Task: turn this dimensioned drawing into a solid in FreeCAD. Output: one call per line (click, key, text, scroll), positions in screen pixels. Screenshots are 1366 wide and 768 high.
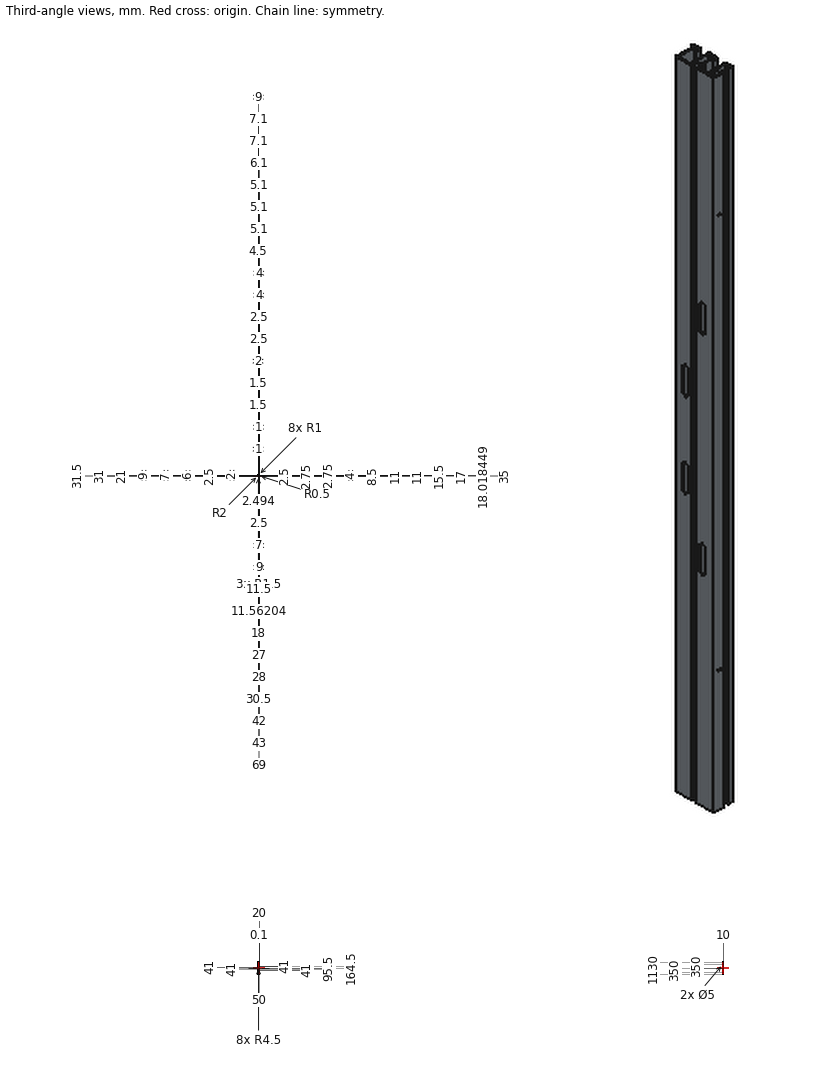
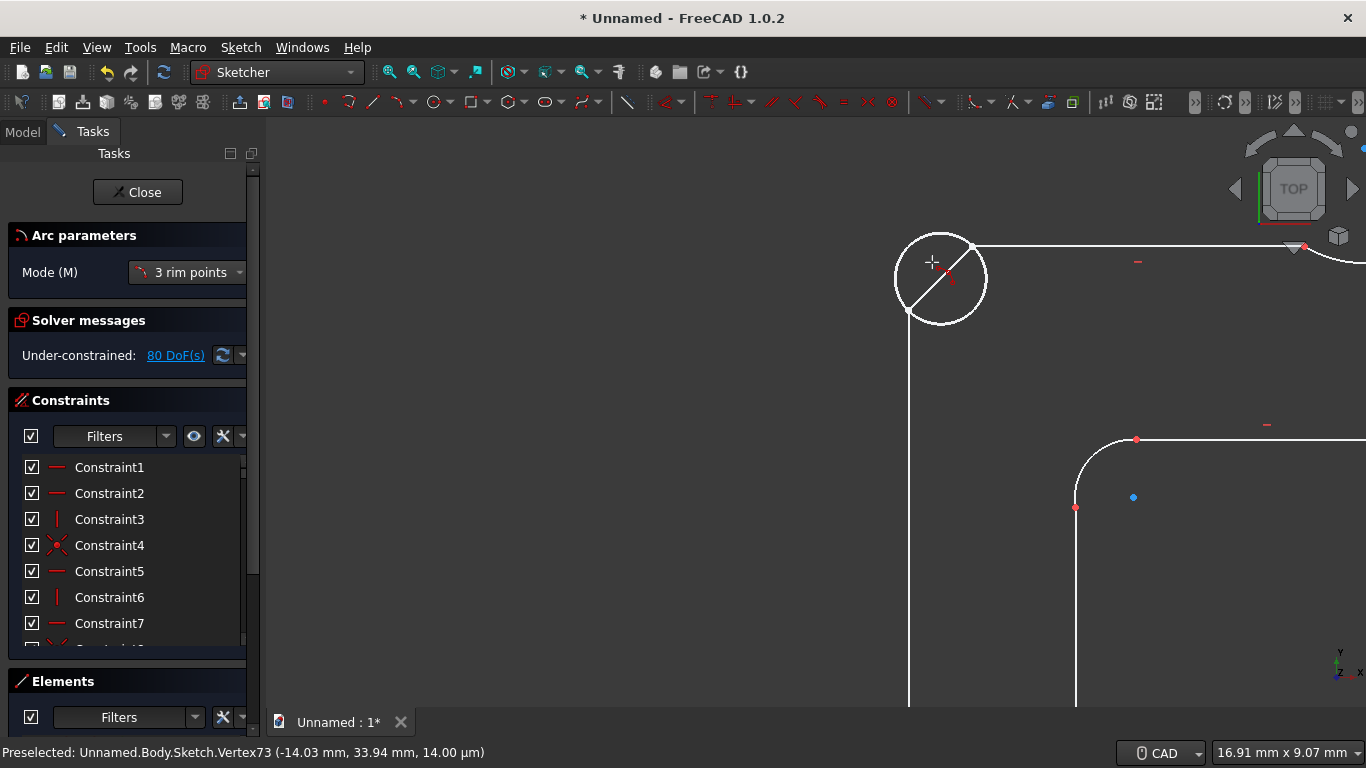
click(929, 261)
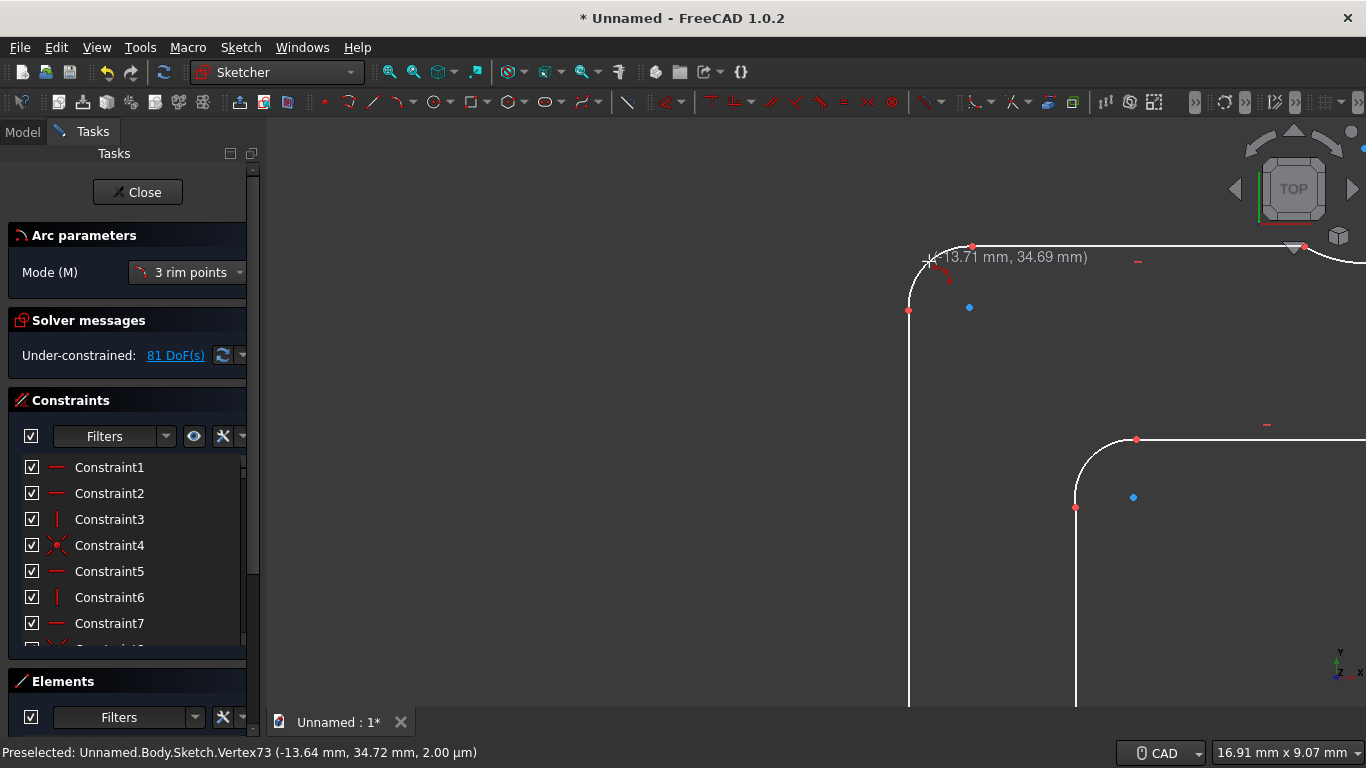
scroll(936, 260, down, 10)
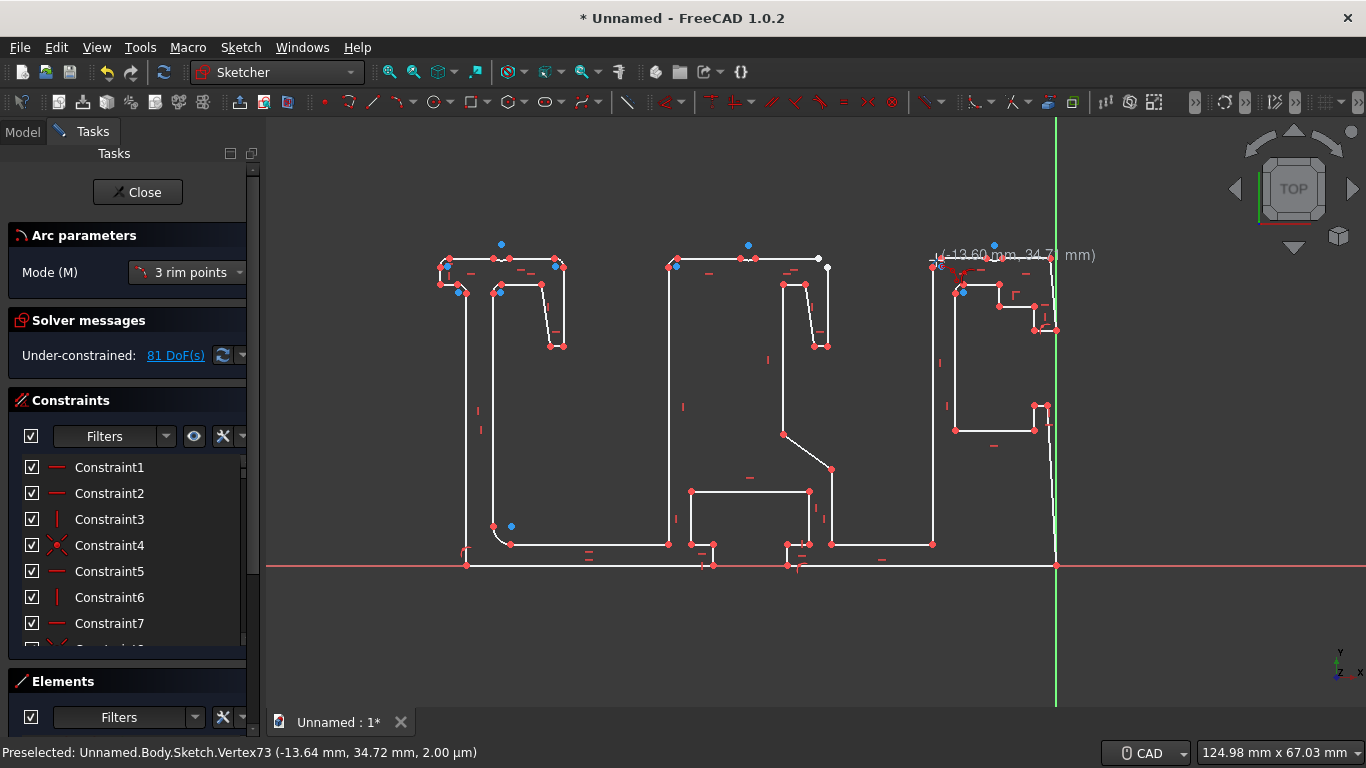
scroll(827, 267, up, 2)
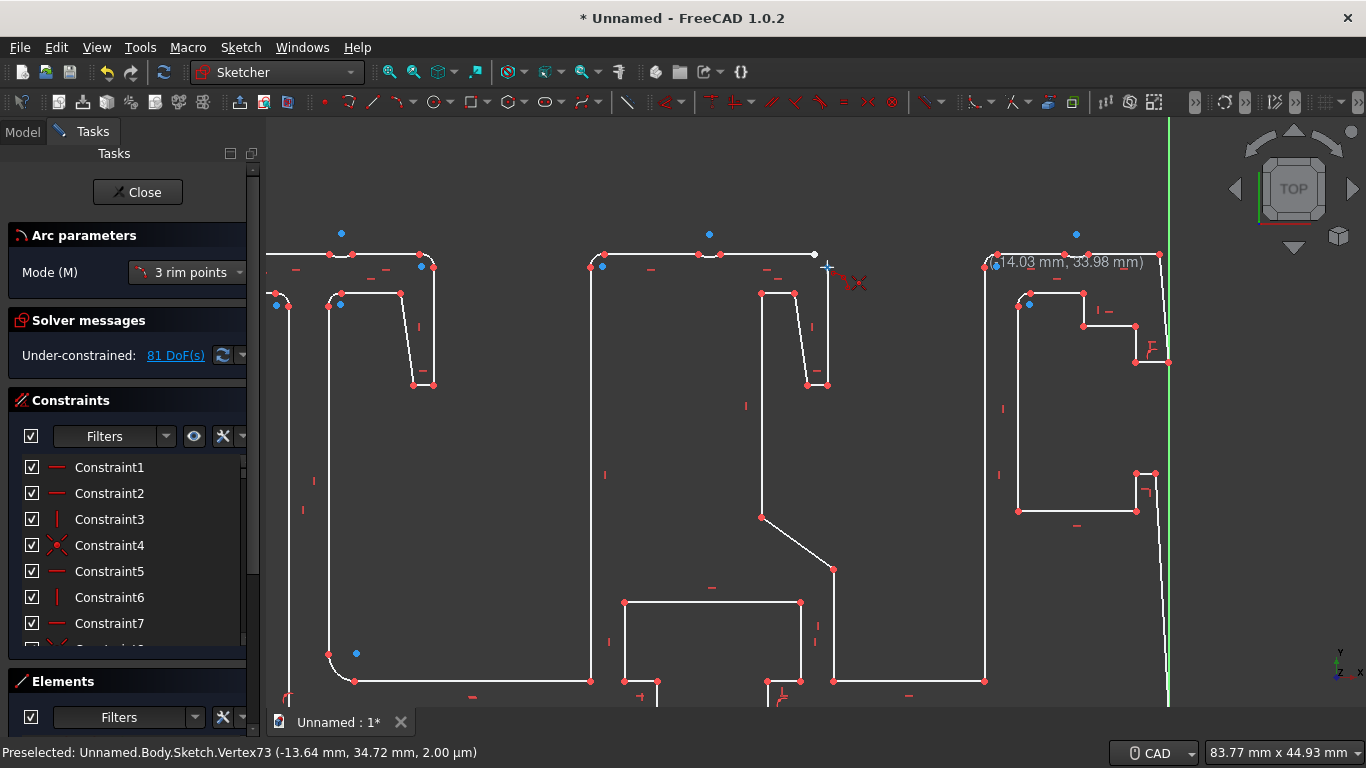
click(828, 267)
click(814, 254)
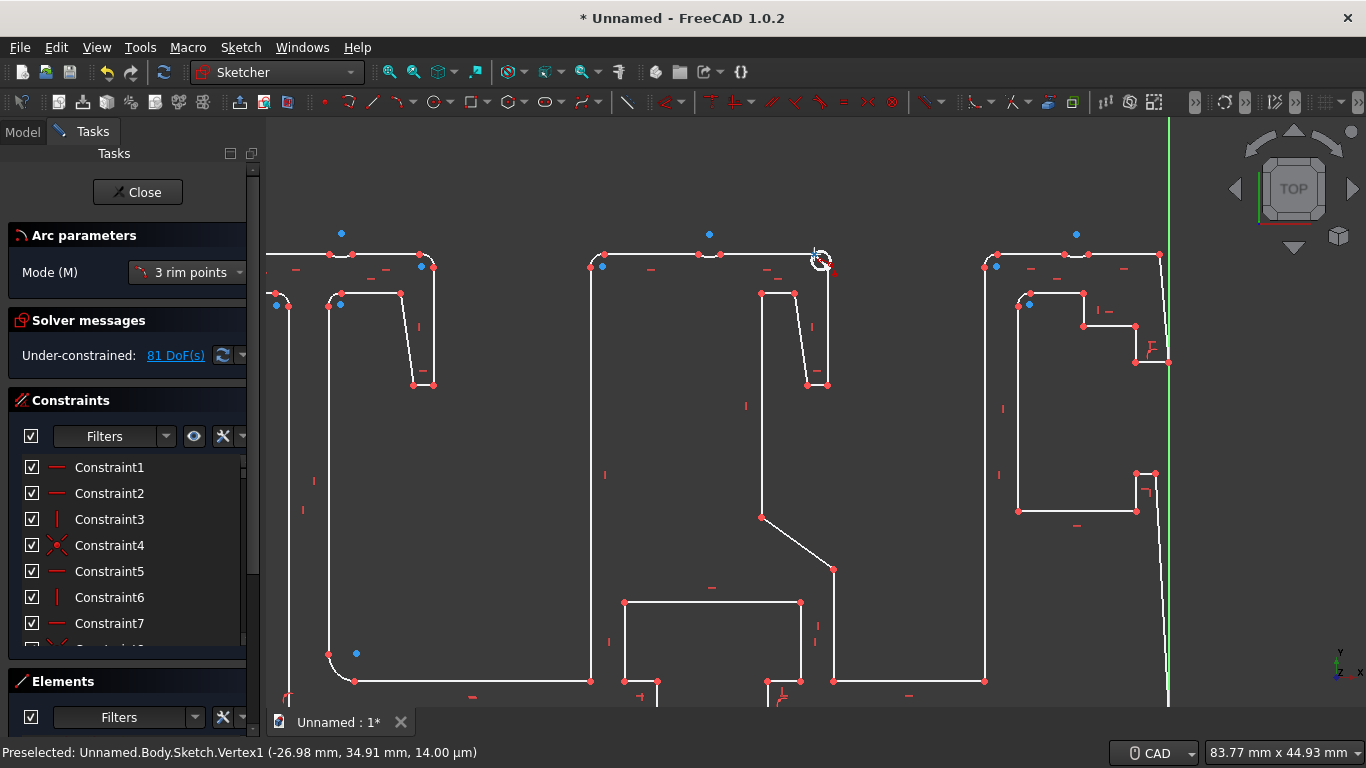
scroll(824, 257, up, 8)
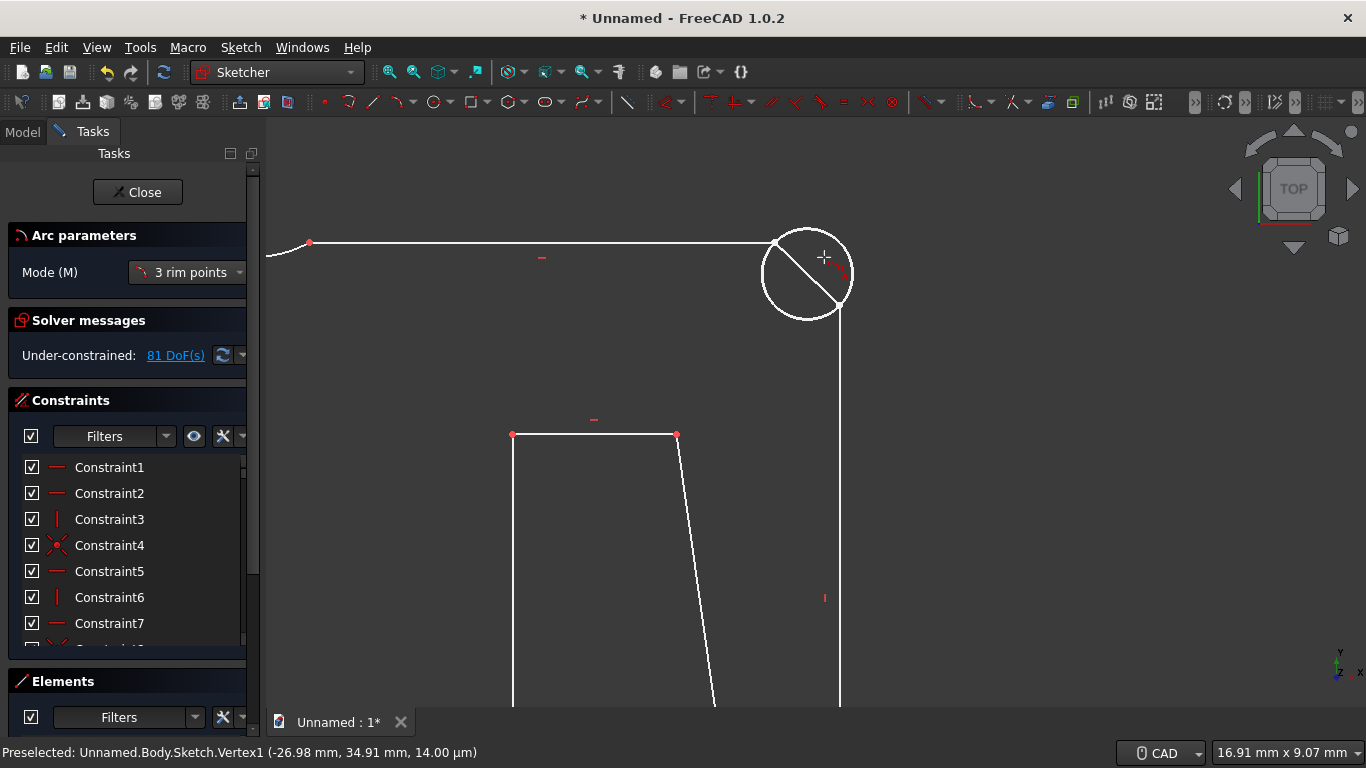
click(820, 256)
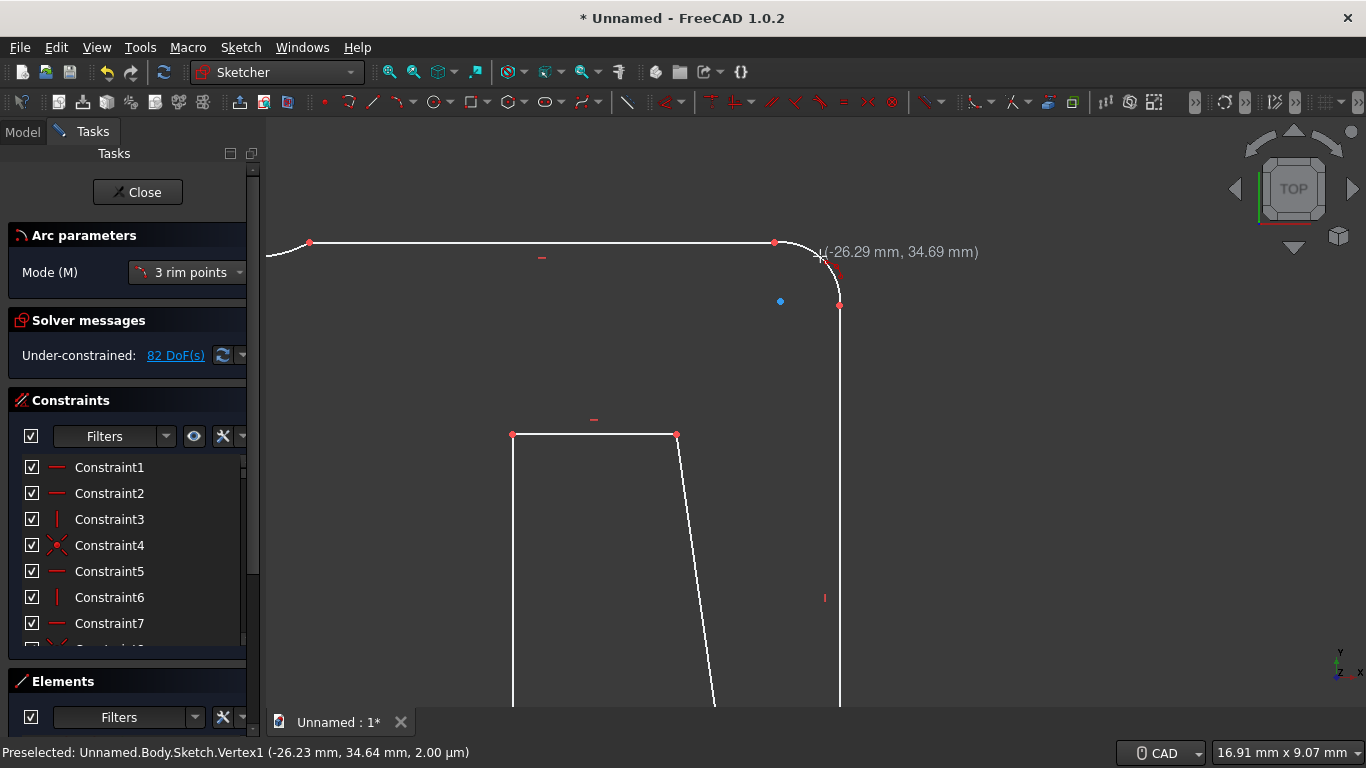
click(472, 102)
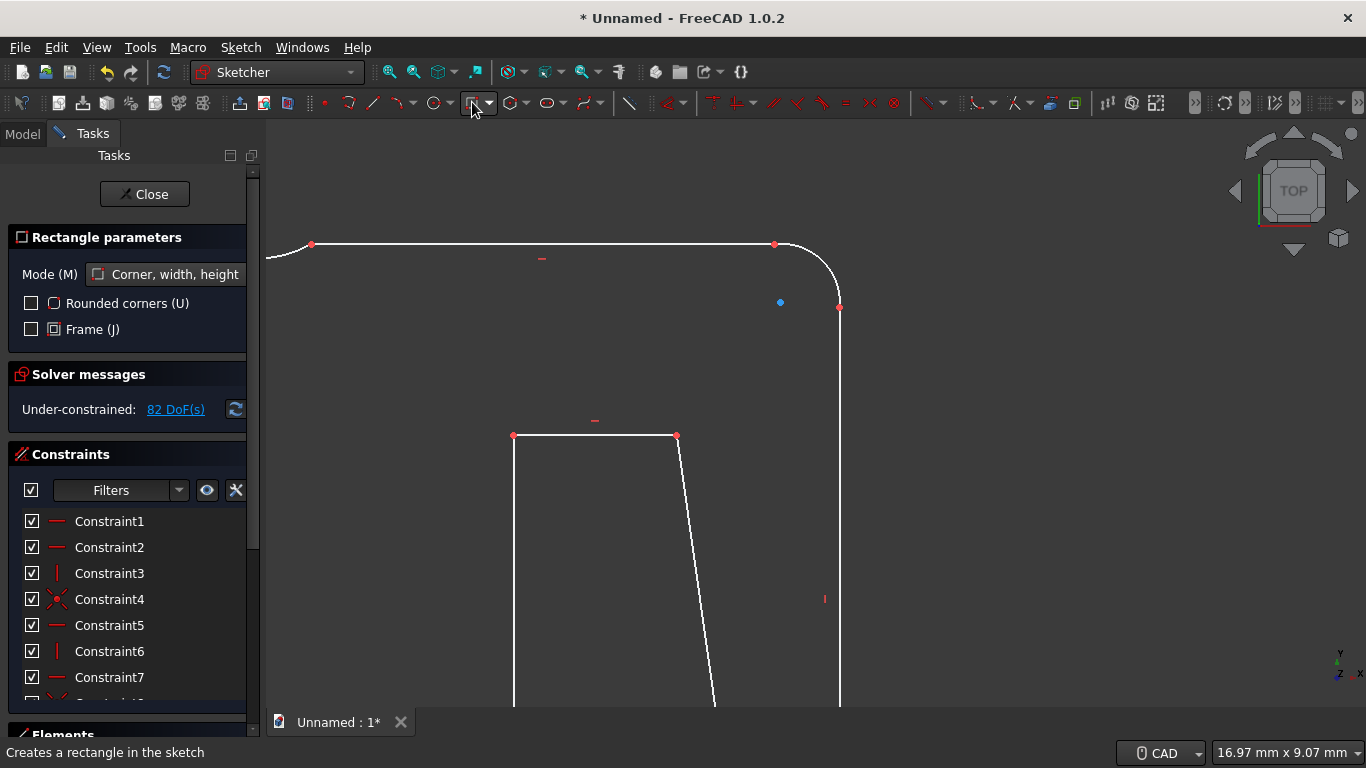
scroll(825, 263, down, 10)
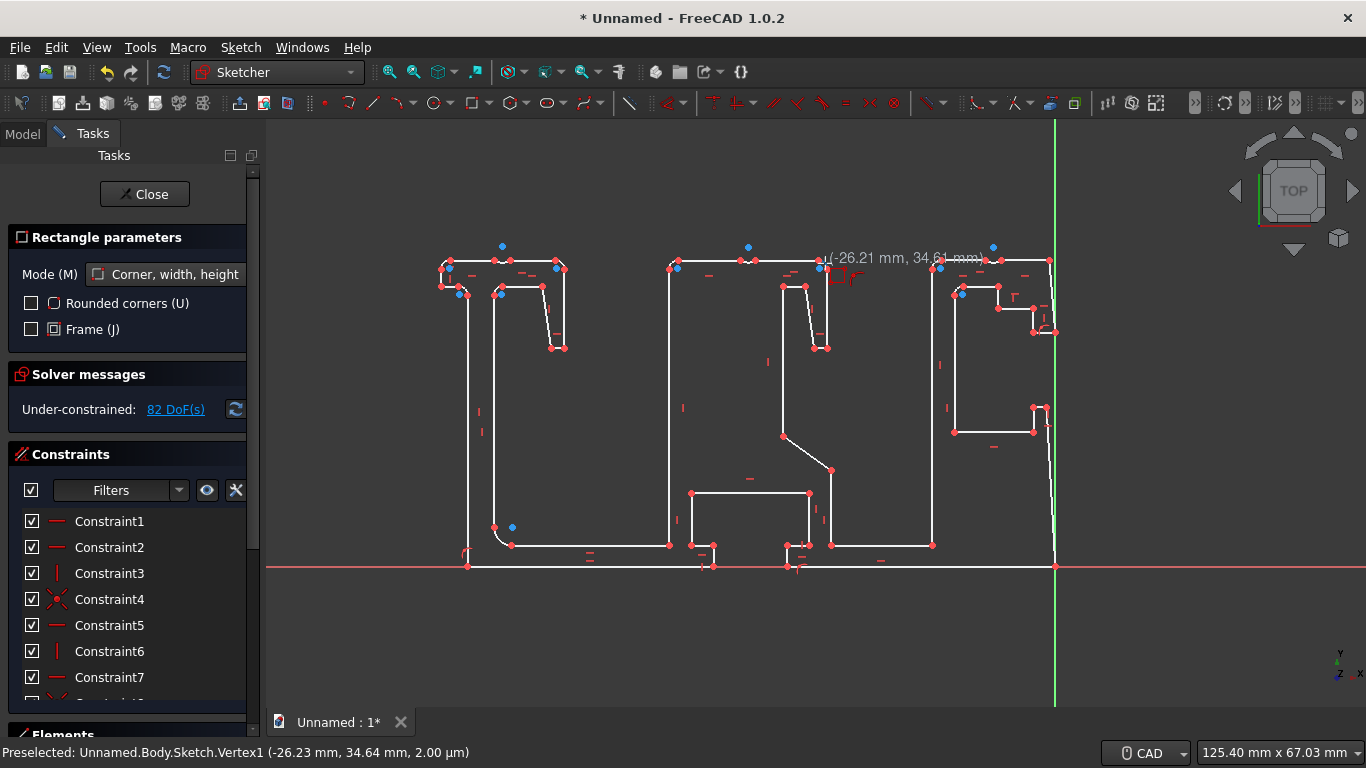
click(954, 448)
click(1033, 545)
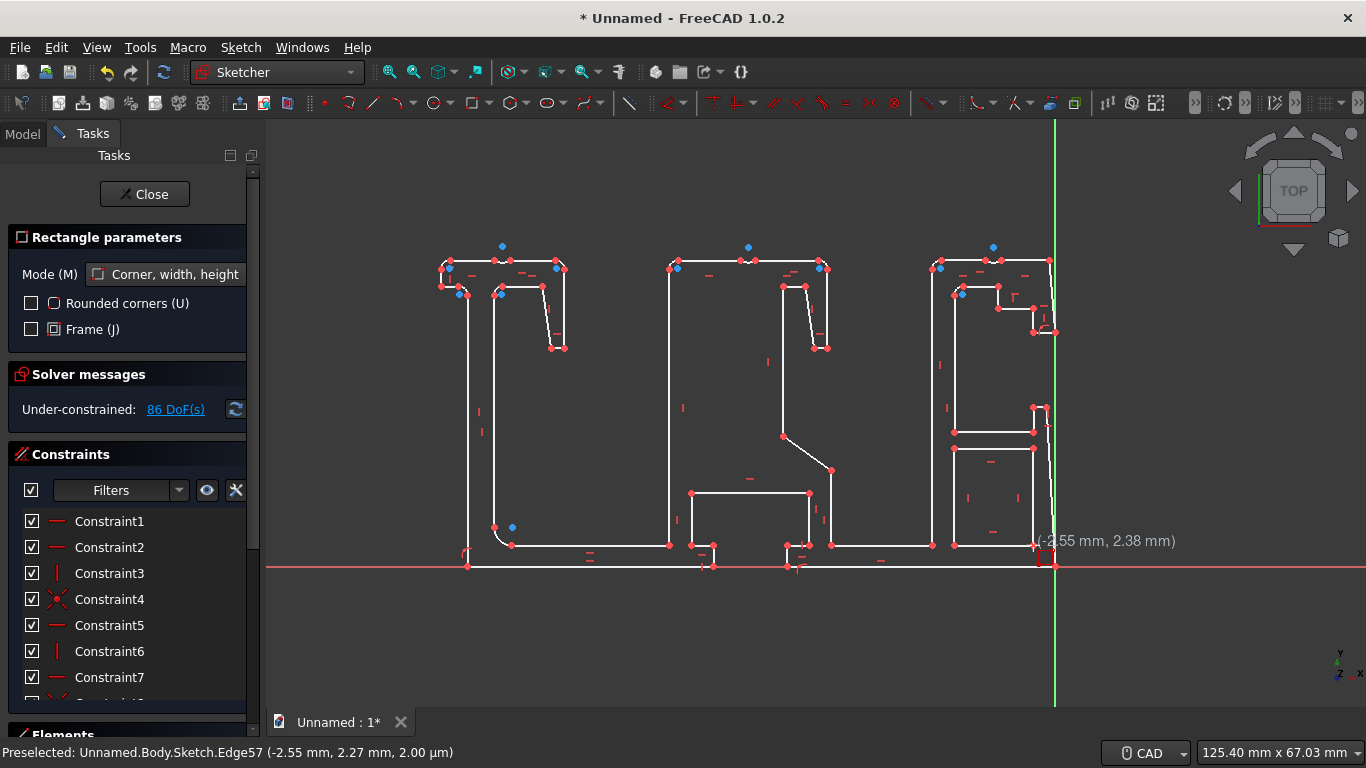
key(g)
key(m)